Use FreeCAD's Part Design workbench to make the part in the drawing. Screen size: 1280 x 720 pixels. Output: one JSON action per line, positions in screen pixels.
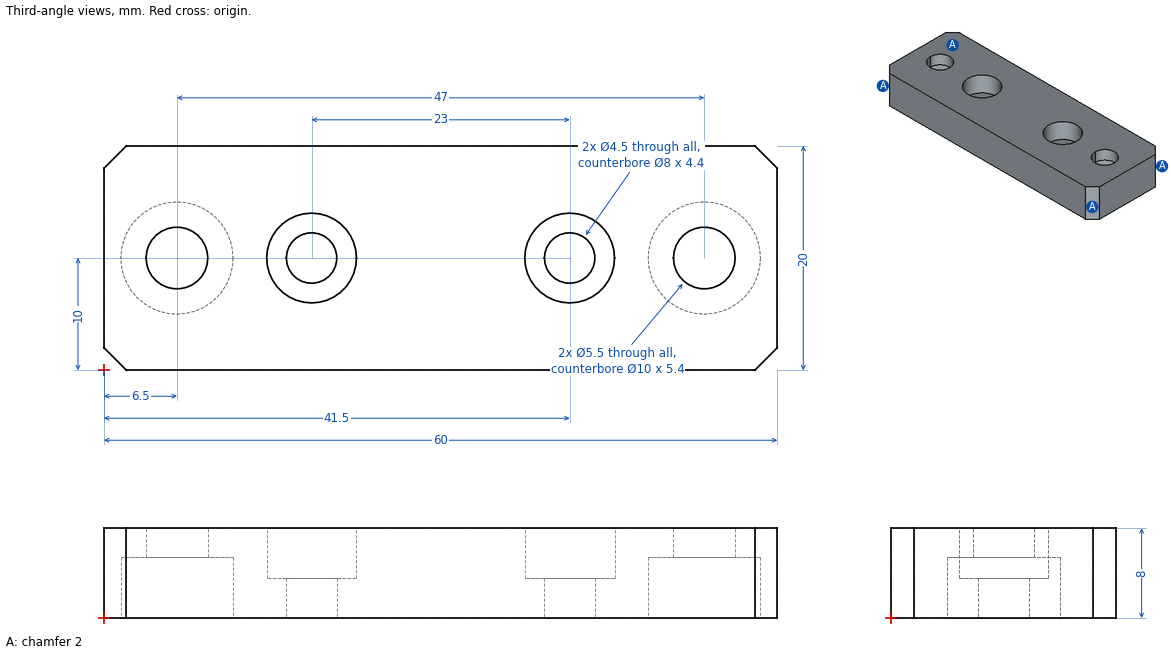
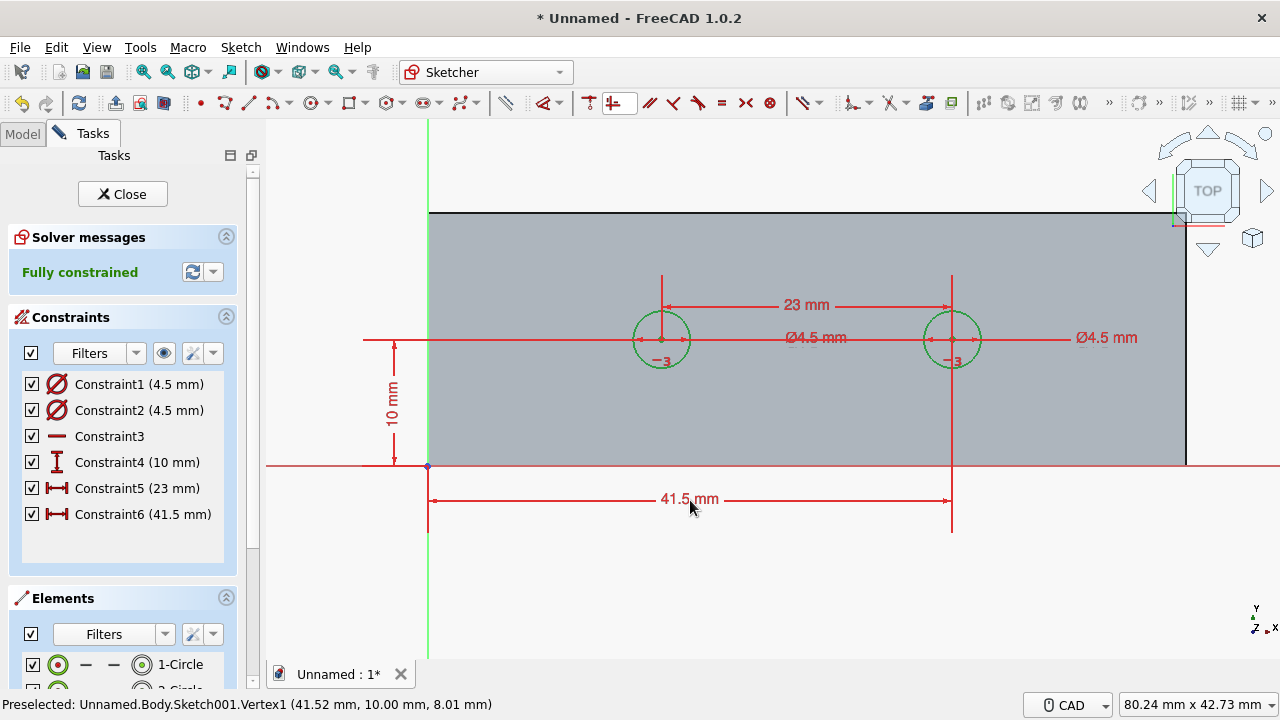
{"action": "left_click", "coordinate": [123, 194]}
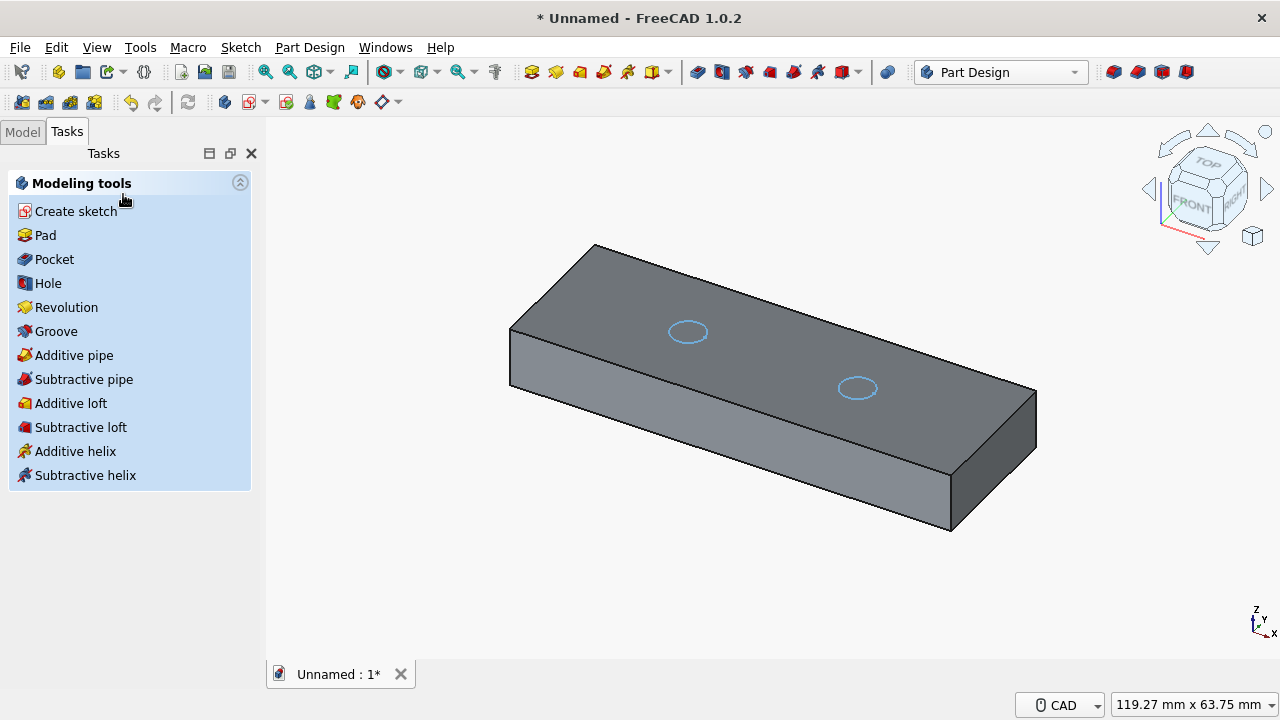
{"action": "left_click", "coordinate": [722, 72]}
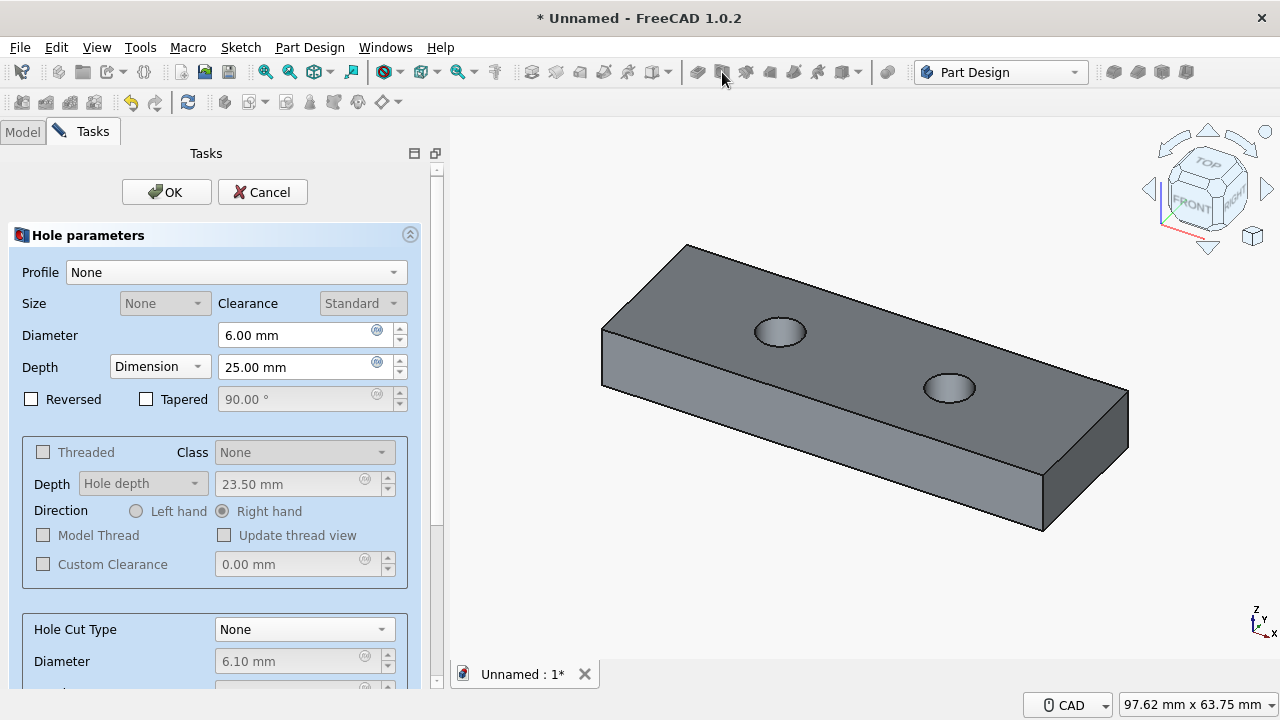
{"action": "triple_click", "coordinate": [305, 335]}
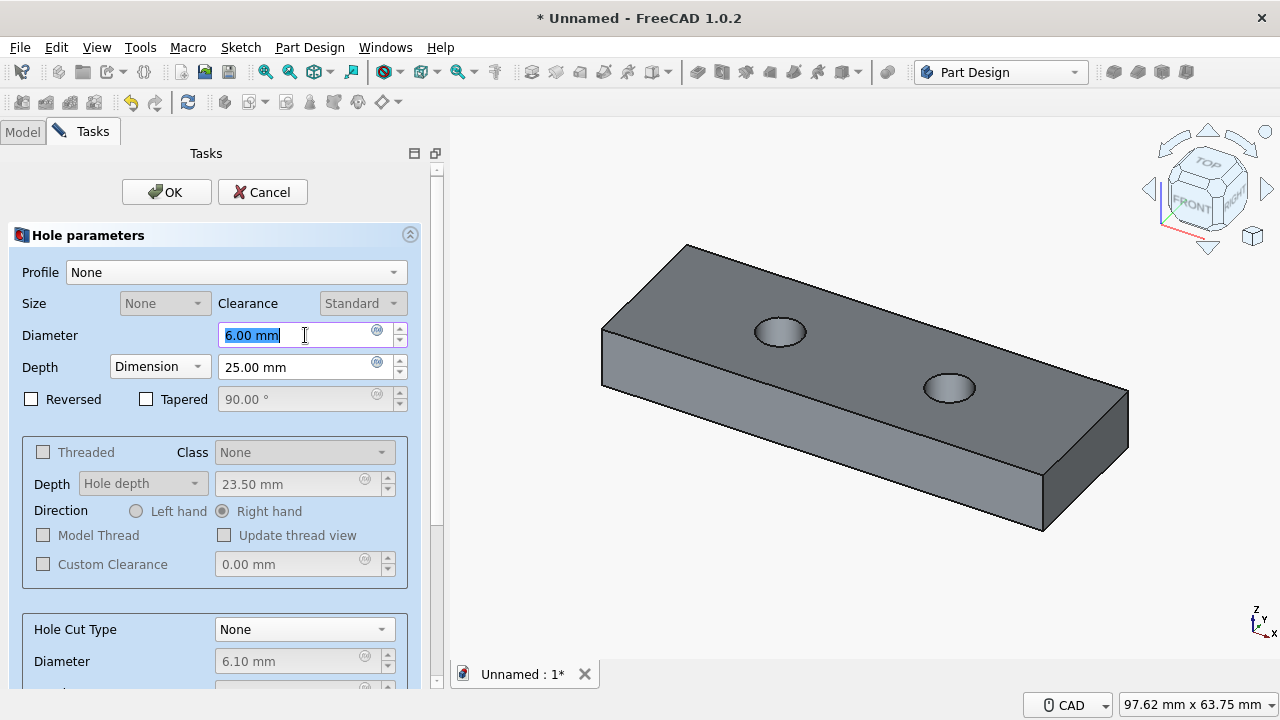
{"action": "type", "text": "4.5"}
{"action": "key", "text": "Tab"}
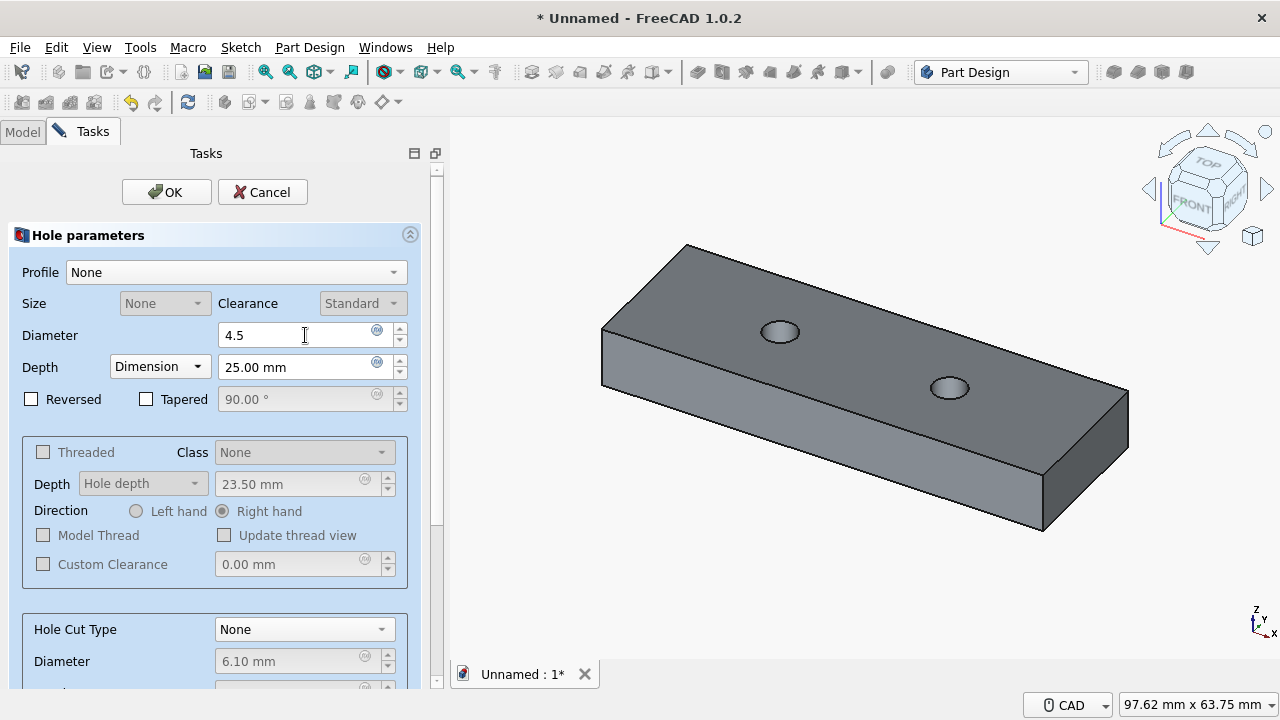
{"action": "left_click", "coordinate": [161, 366]}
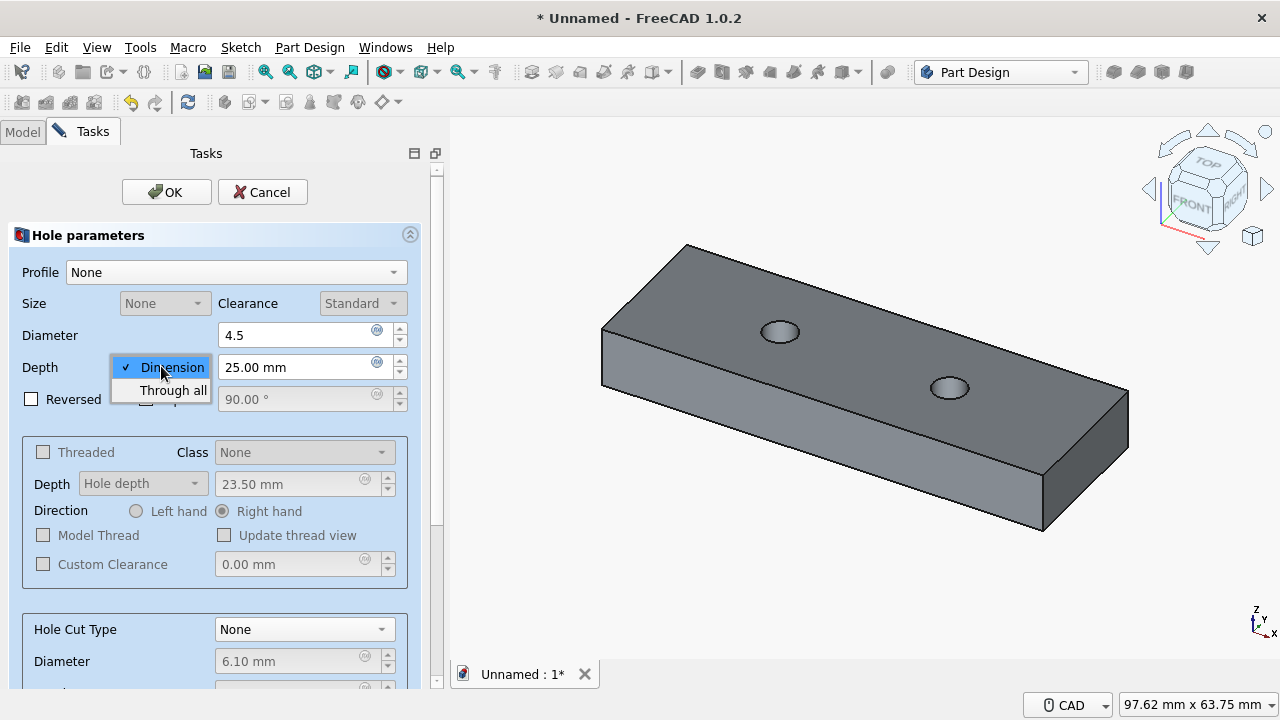
{"action": "left_click", "coordinate": [160, 390]}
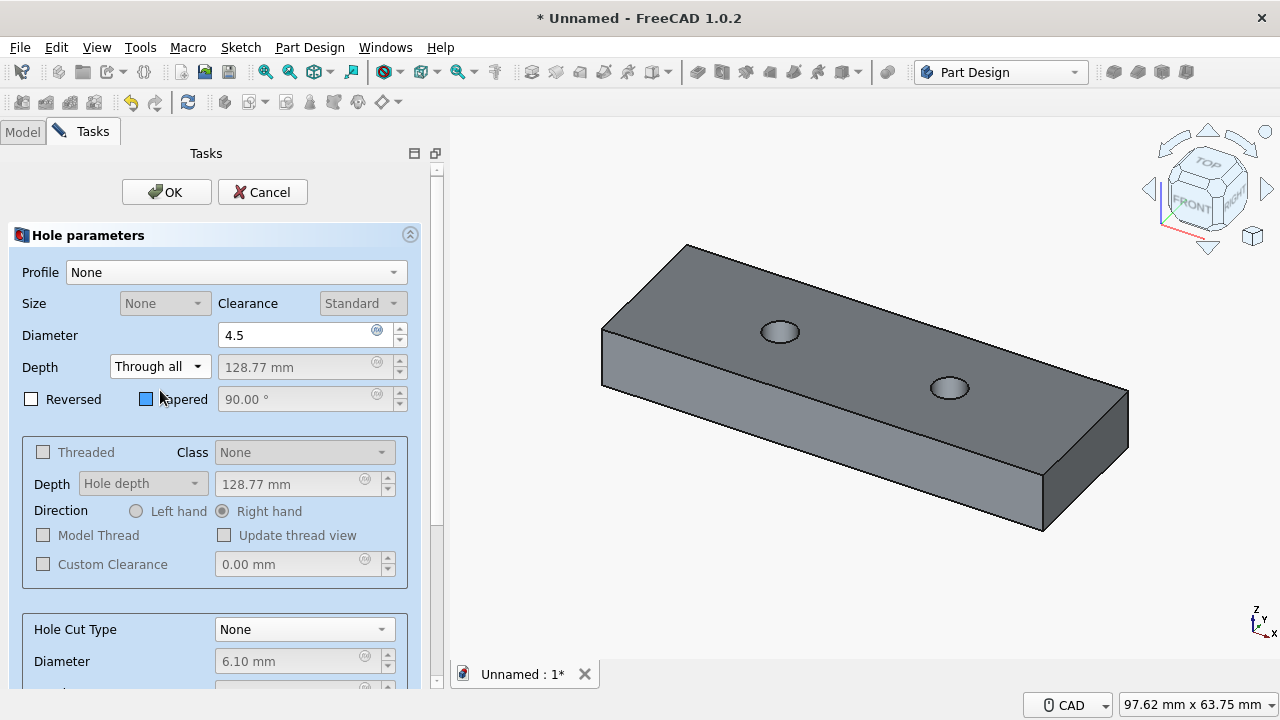
{"action": "left_click", "coordinate": [306, 630]}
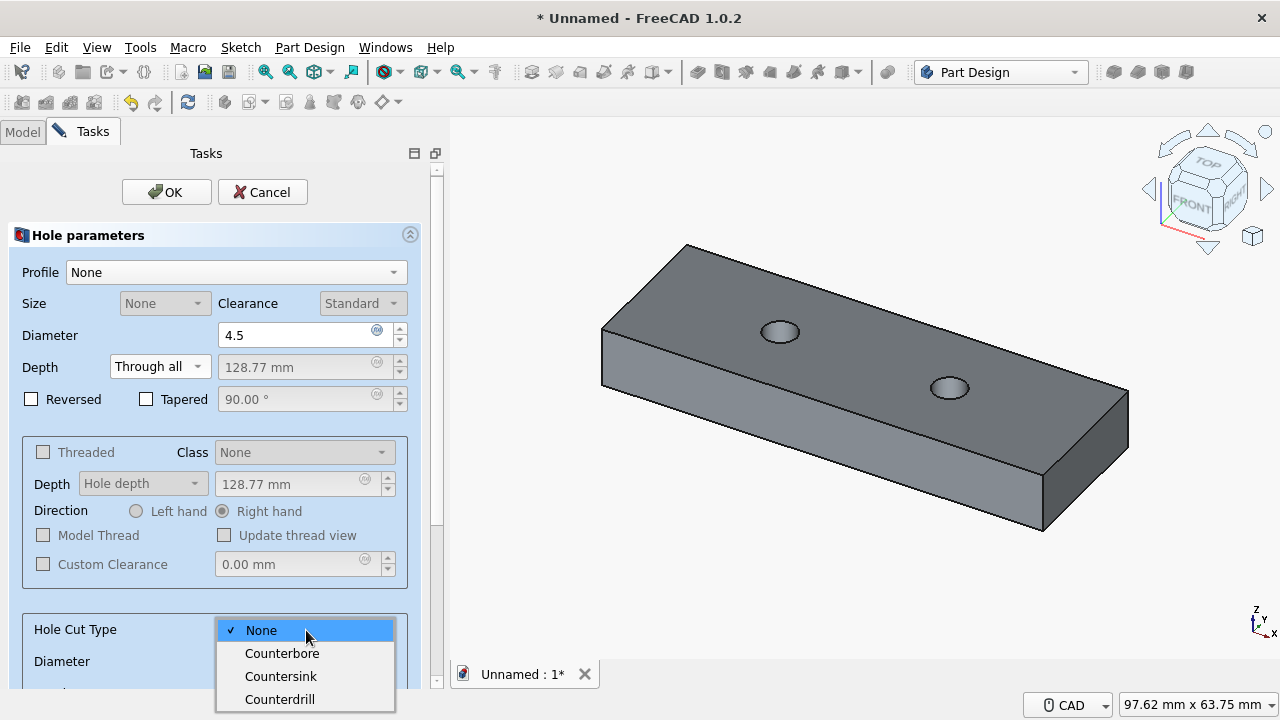
{"action": "left_click", "coordinate": [304, 654]}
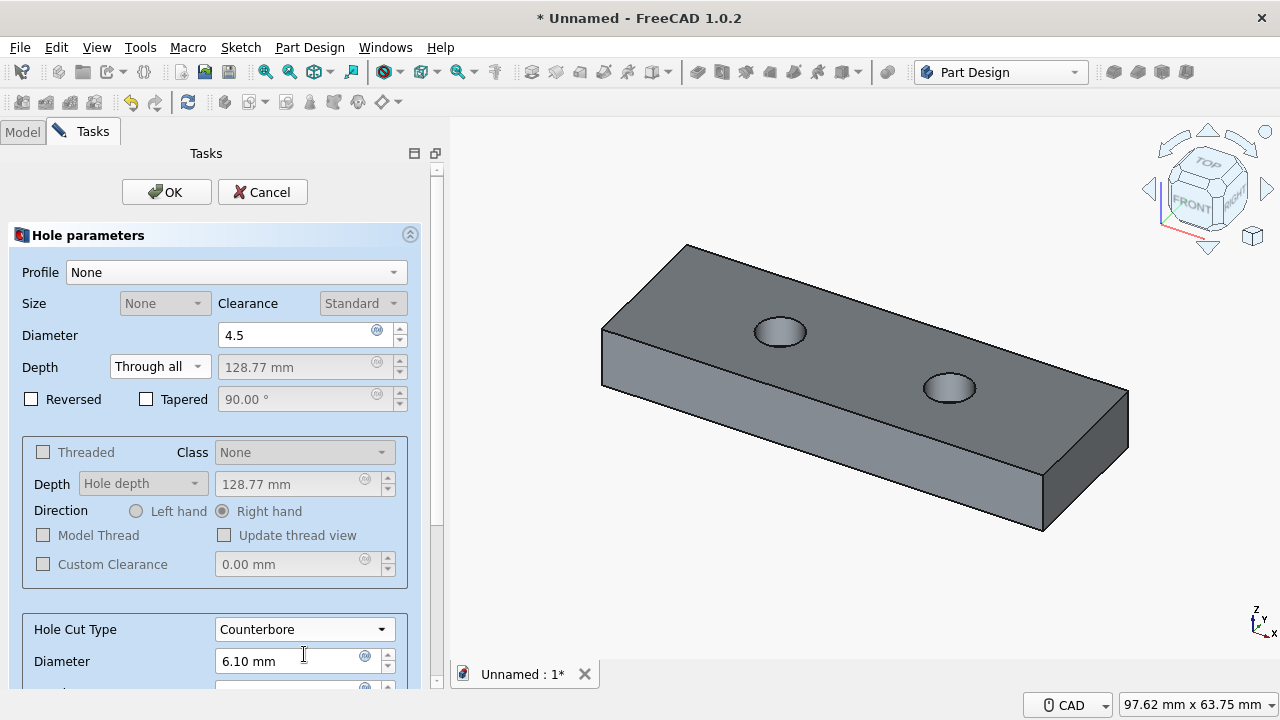
{"action": "triple_click", "coordinate": [298, 661]}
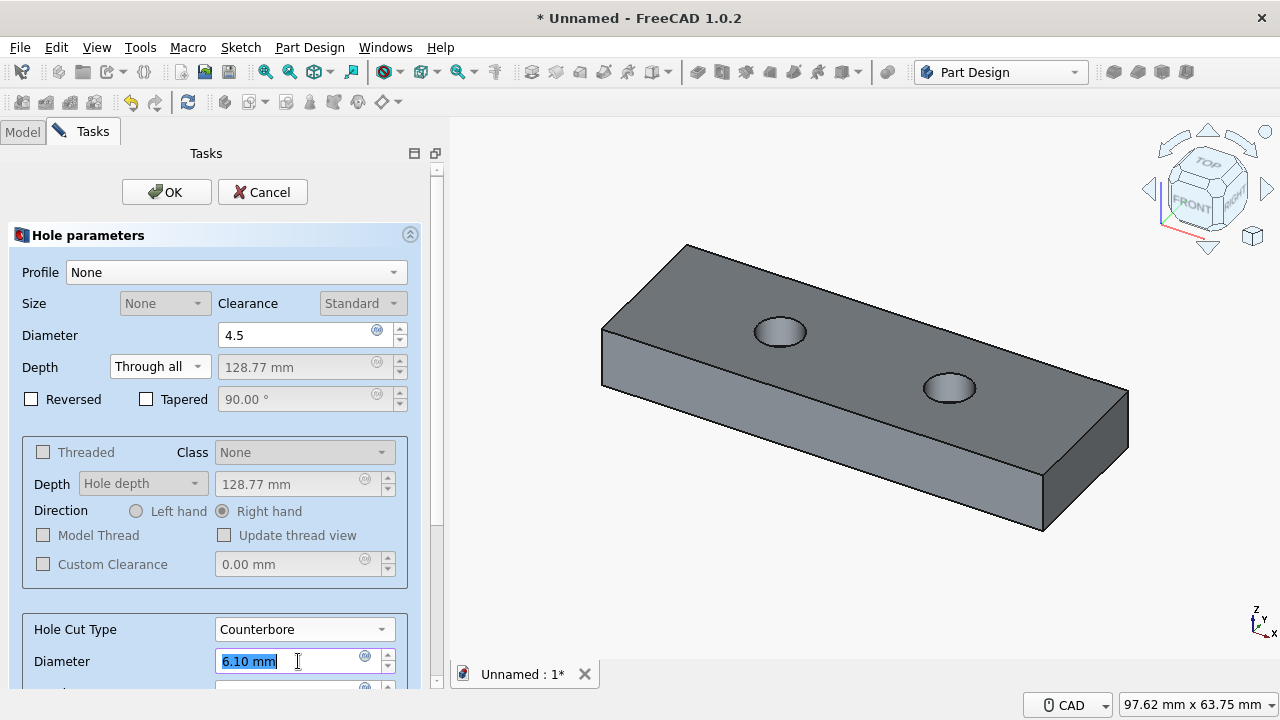
{"action": "type", "text": "8"}
{"action": "key", "text": "Tab"}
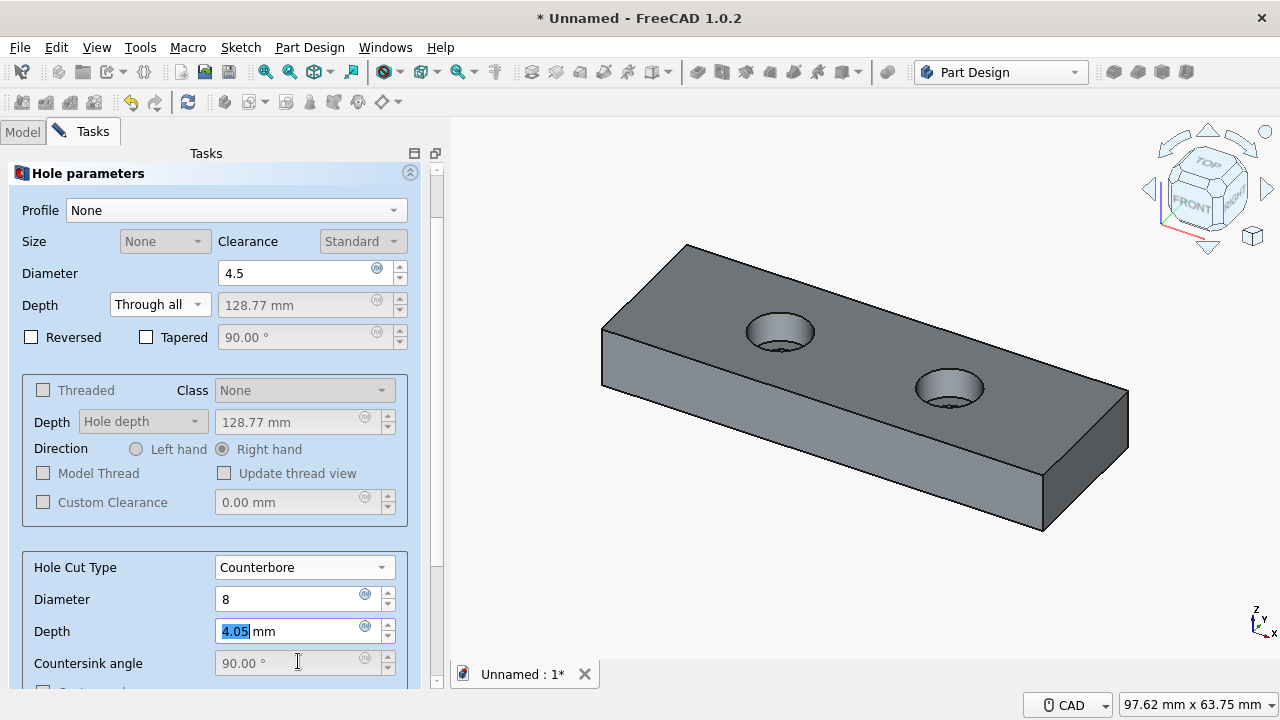
{"action": "type", "text": "4.4"}
{"action": "key", "text": "Tab"}